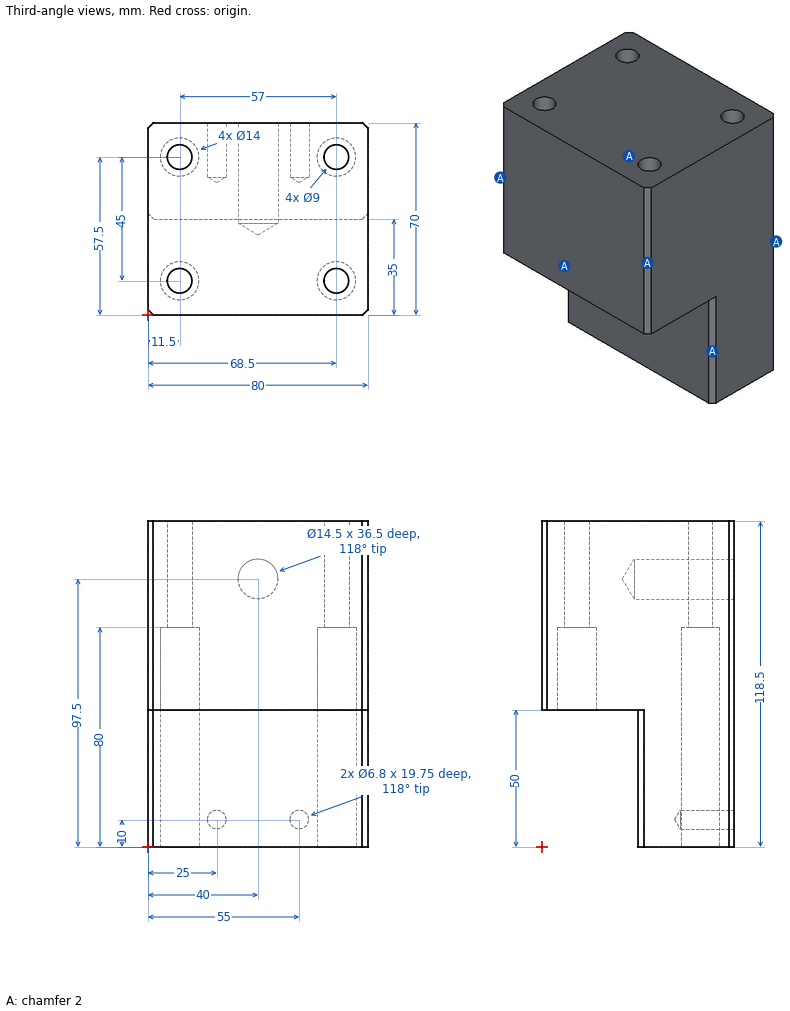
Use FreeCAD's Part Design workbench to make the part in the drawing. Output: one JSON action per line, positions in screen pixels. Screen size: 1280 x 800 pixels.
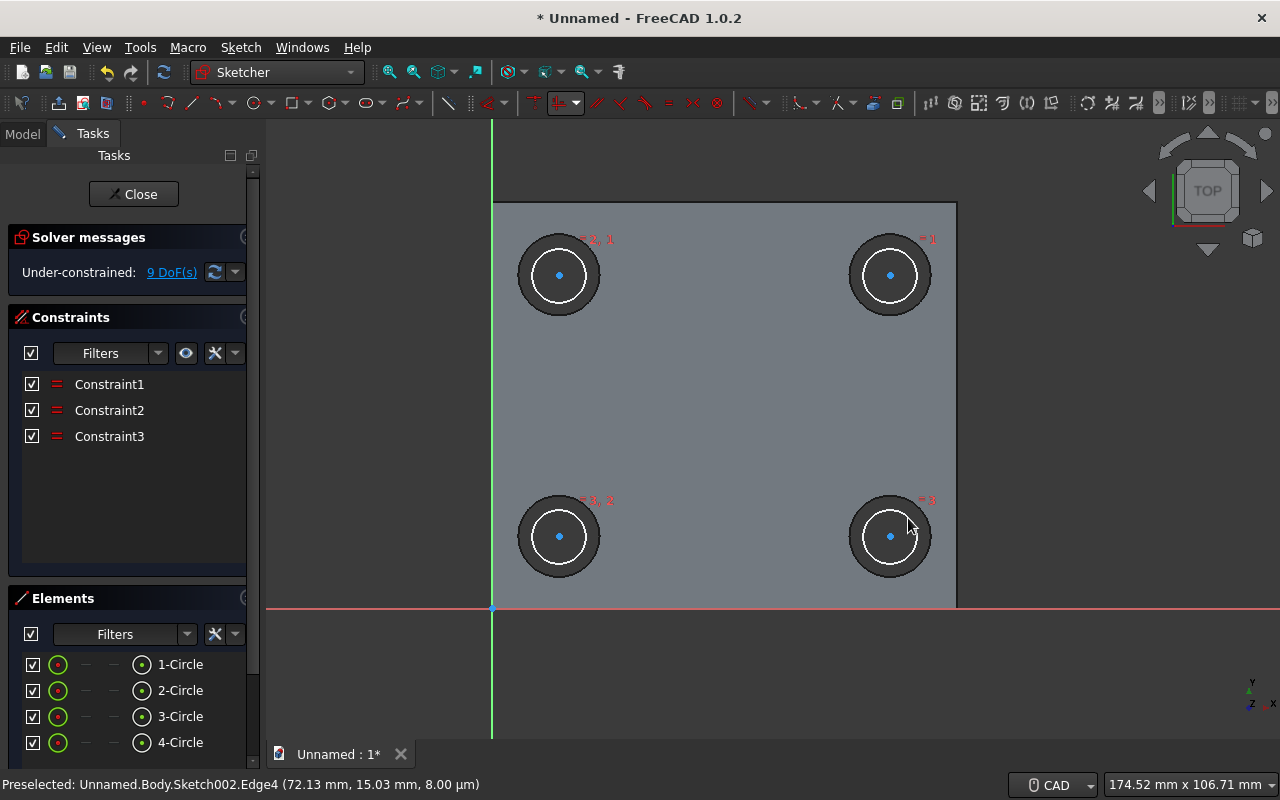
{"action": "left_click", "coordinate": [890, 276]}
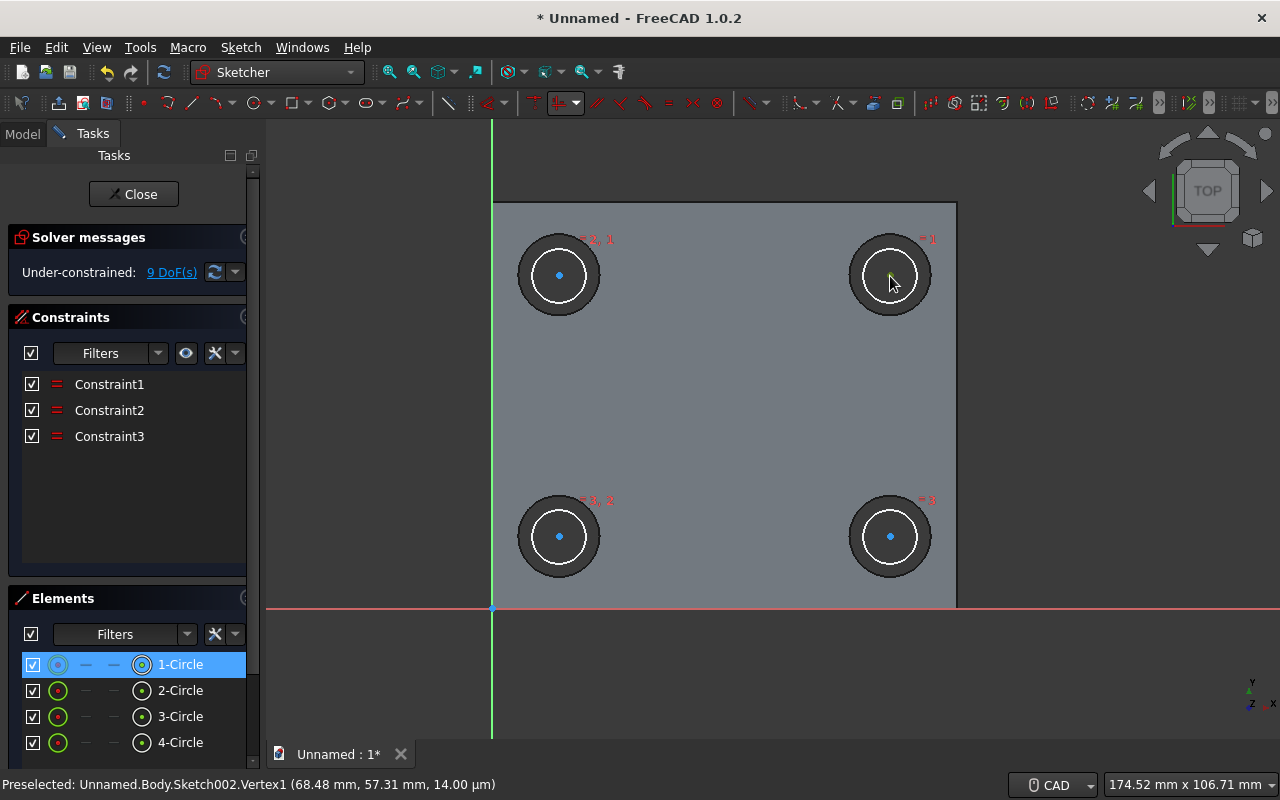
{"action": "left_click", "coordinate": [559, 276]}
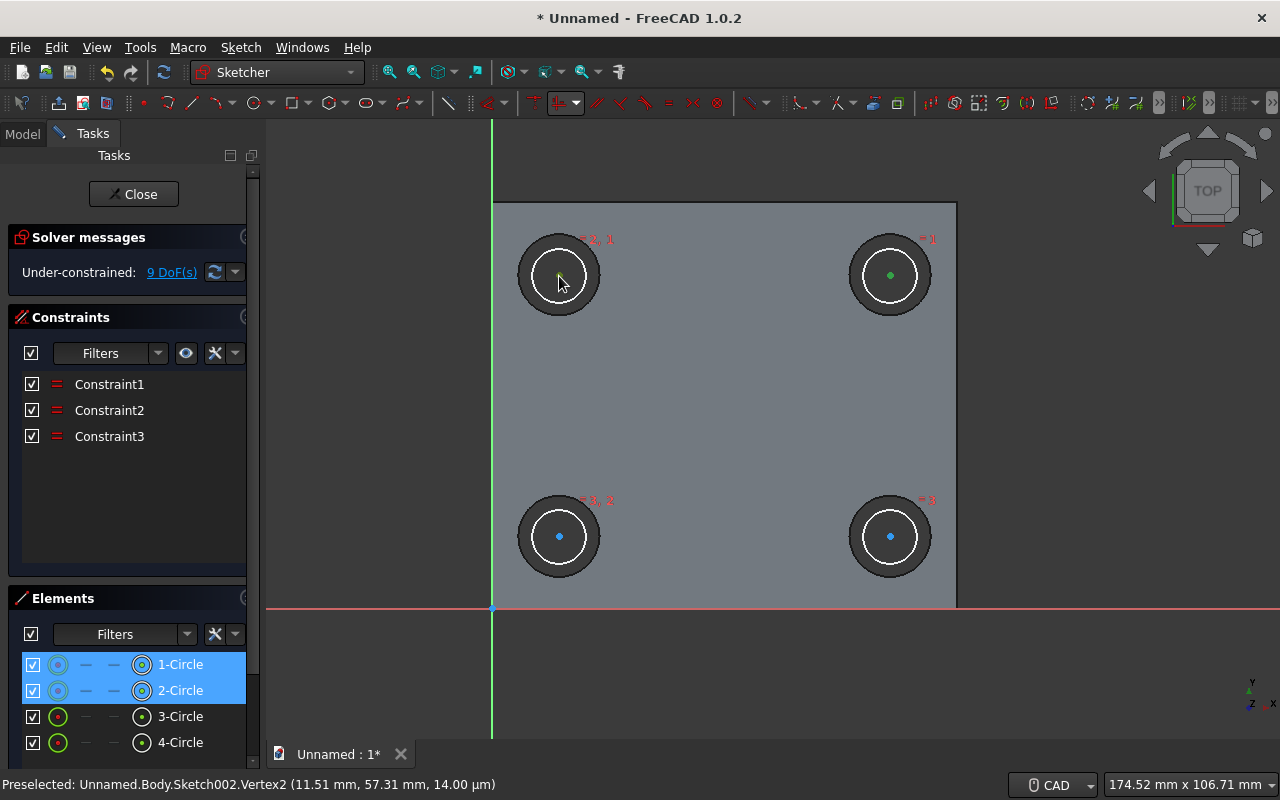
{"action": "key", "text": "h"}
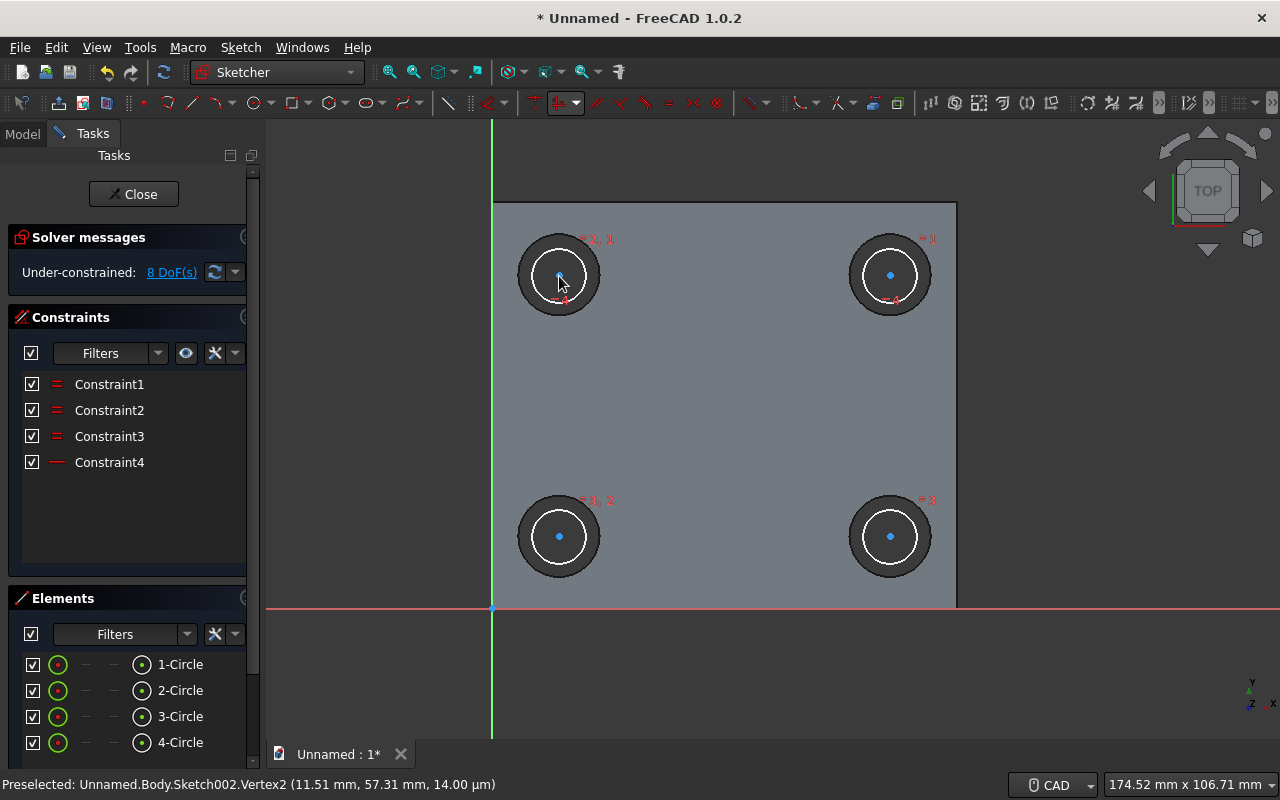
{"action": "left_click", "coordinate": [559, 276]}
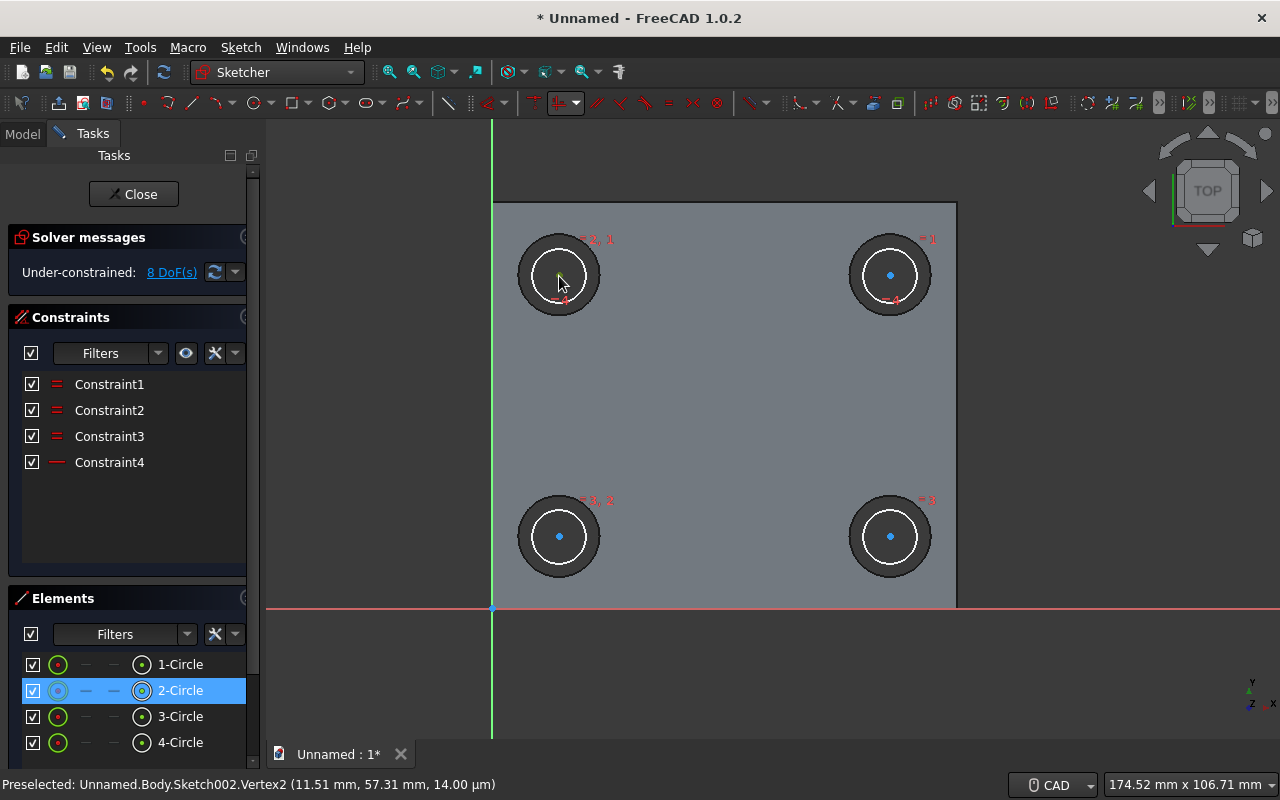
{"action": "left_click", "coordinate": [559, 537]}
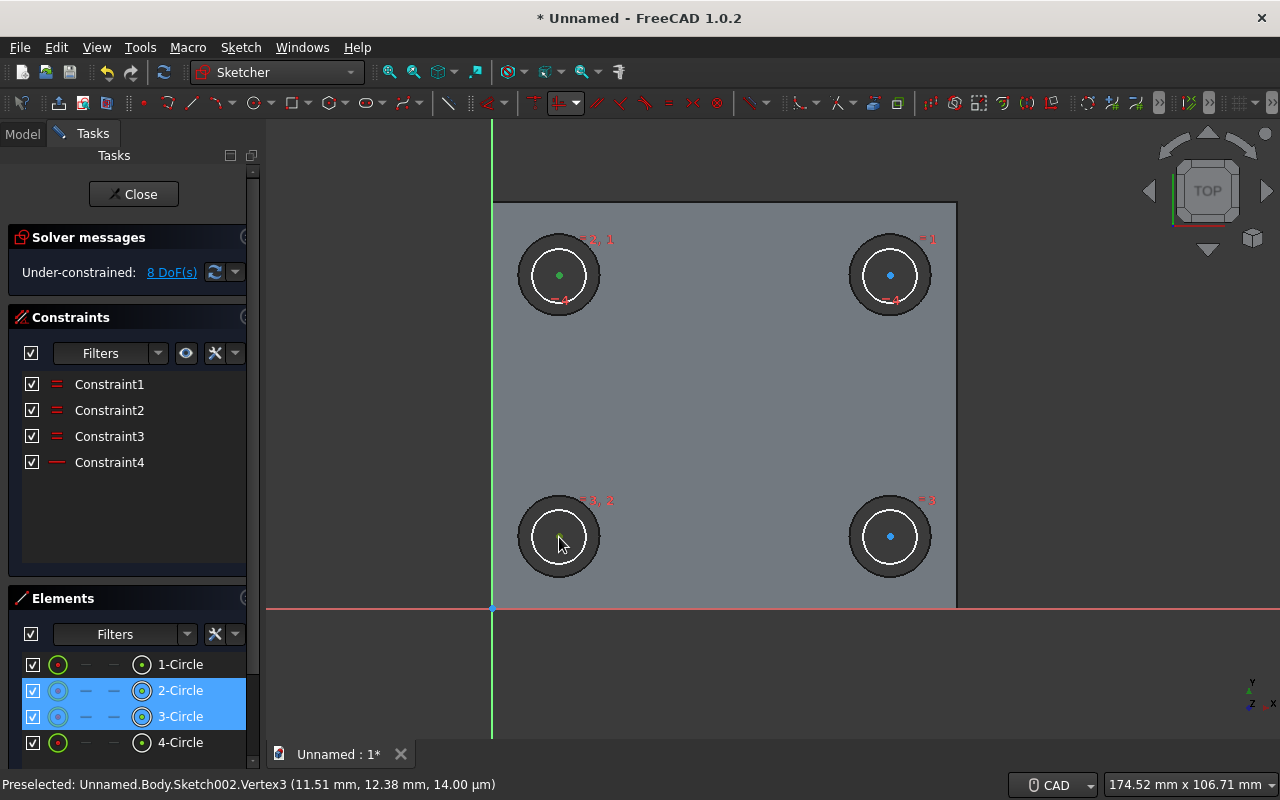
{"action": "key", "text": "v"}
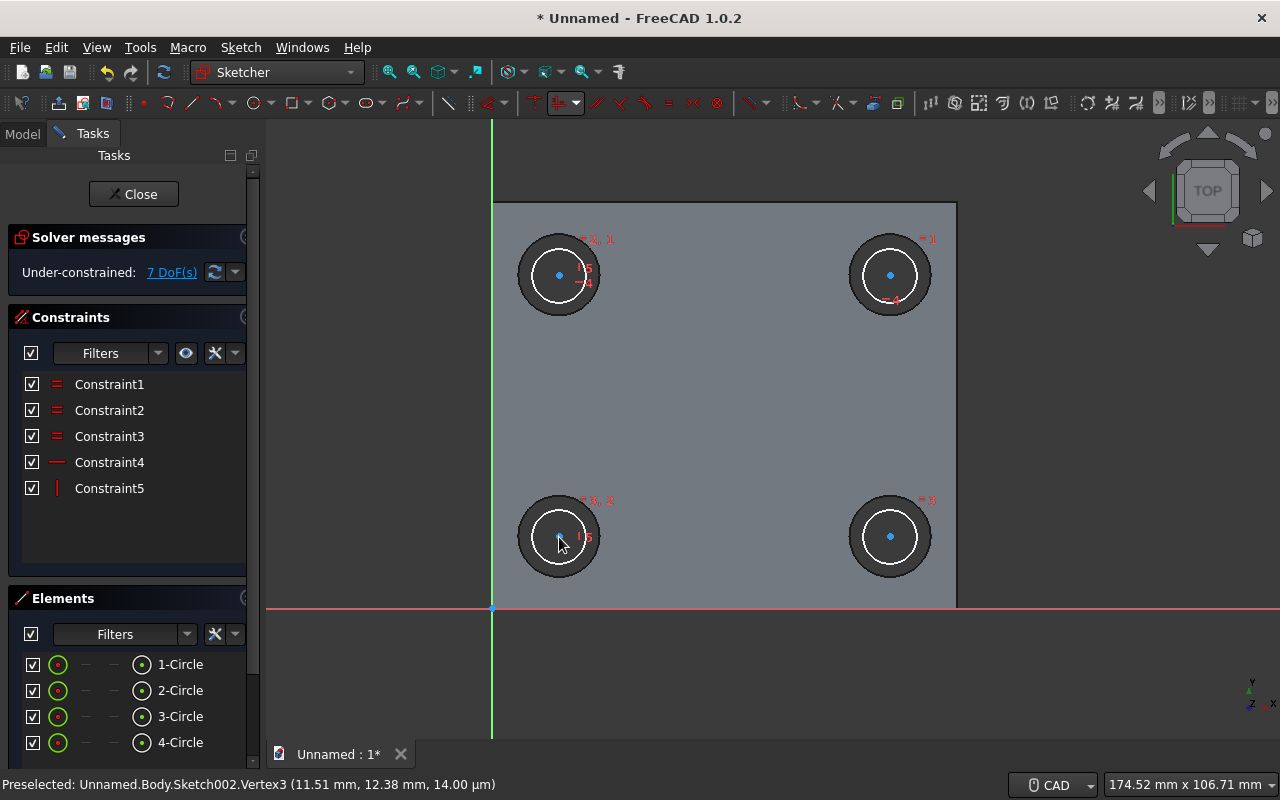
{"action": "left_click", "coordinate": [890, 276]}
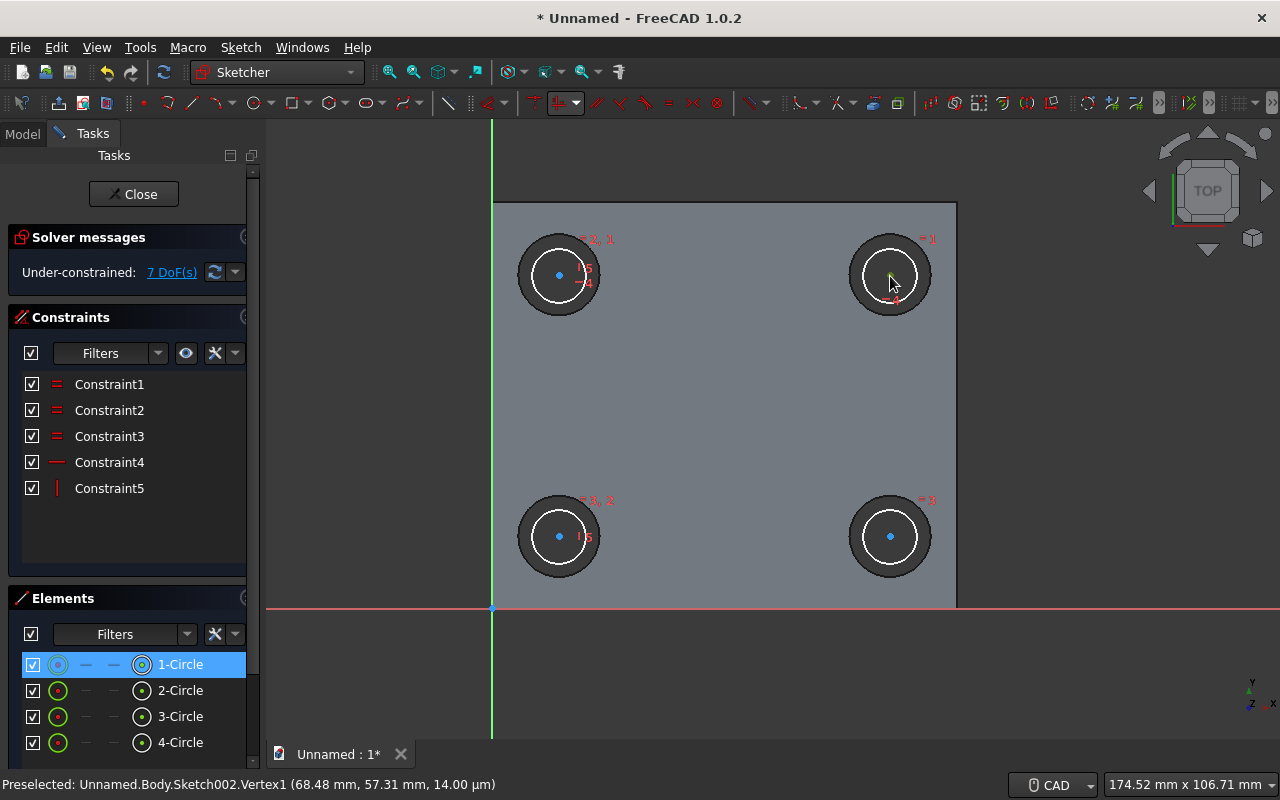
{"action": "left_click", "coordinate": [890, 537]}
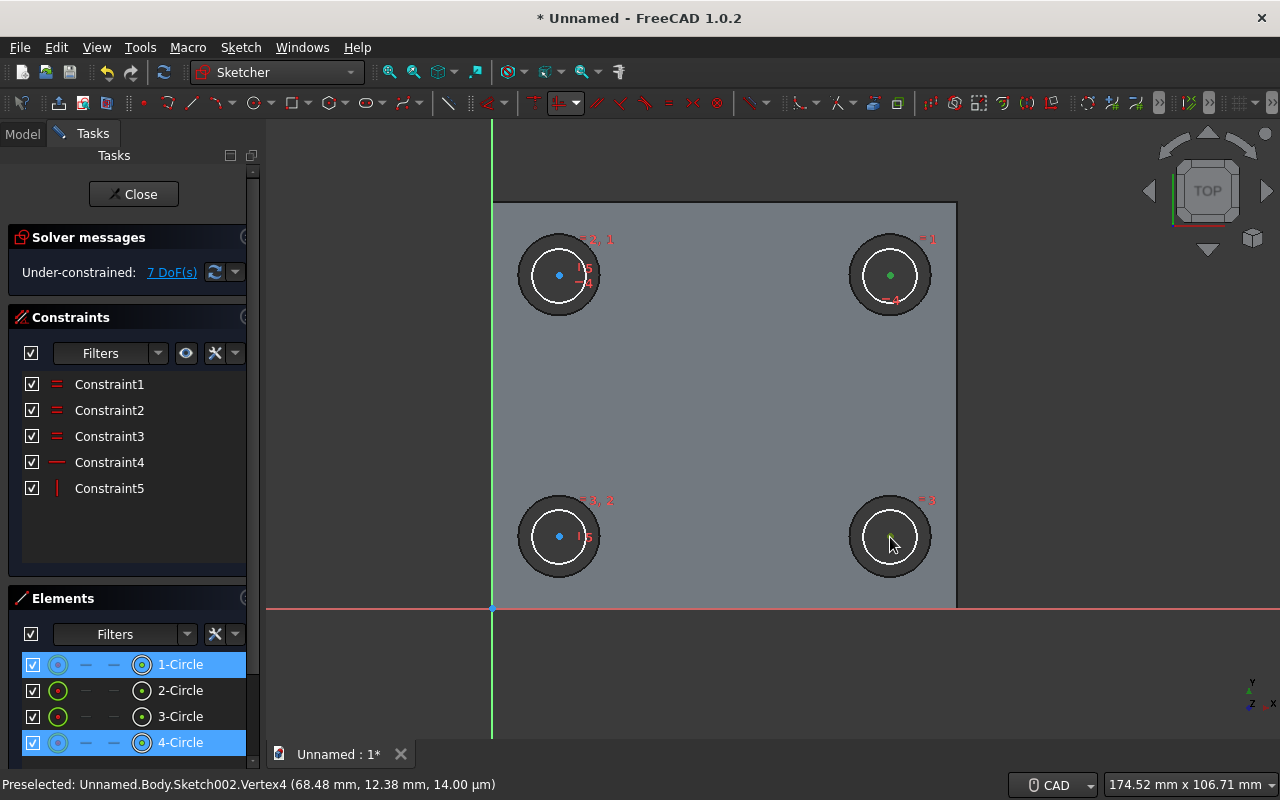
{"action": "left_click", "coordinate": [578, 104]}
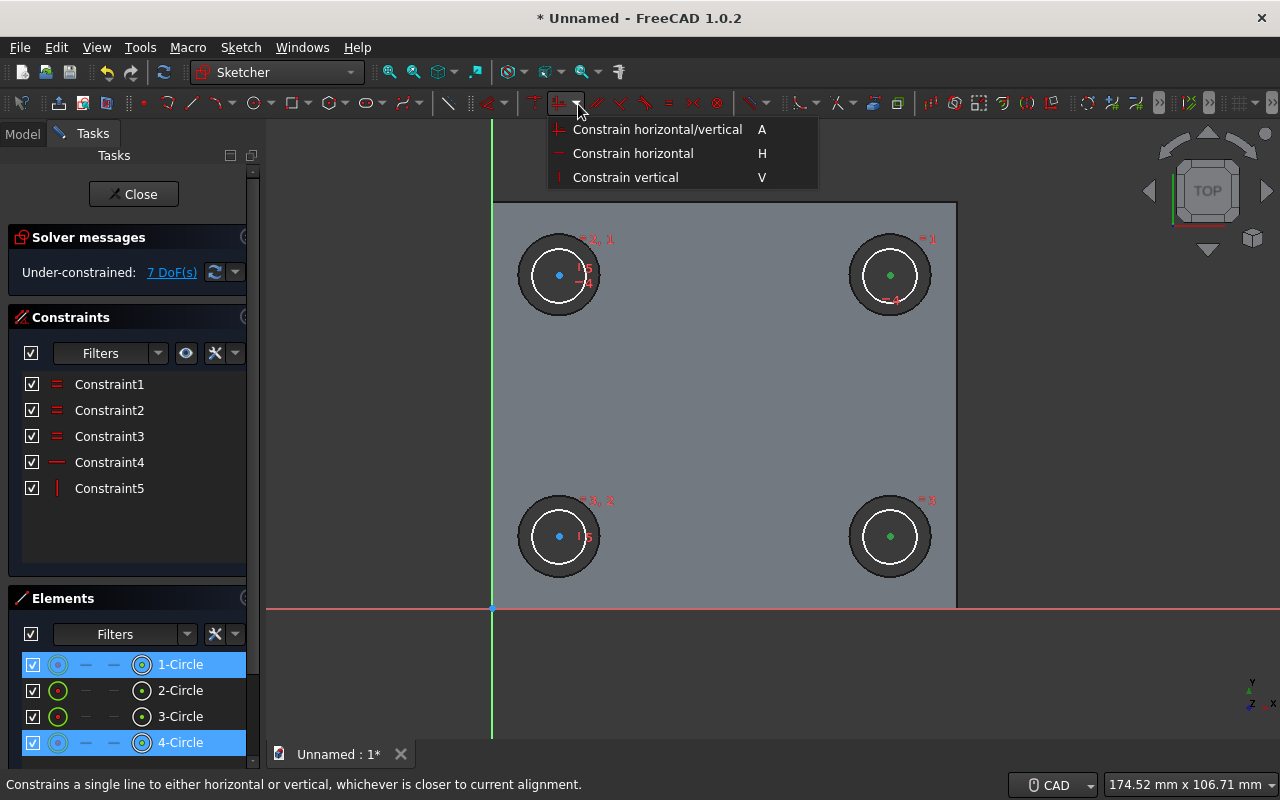
{"action": "left_click", "coordinate": [683, 177]}